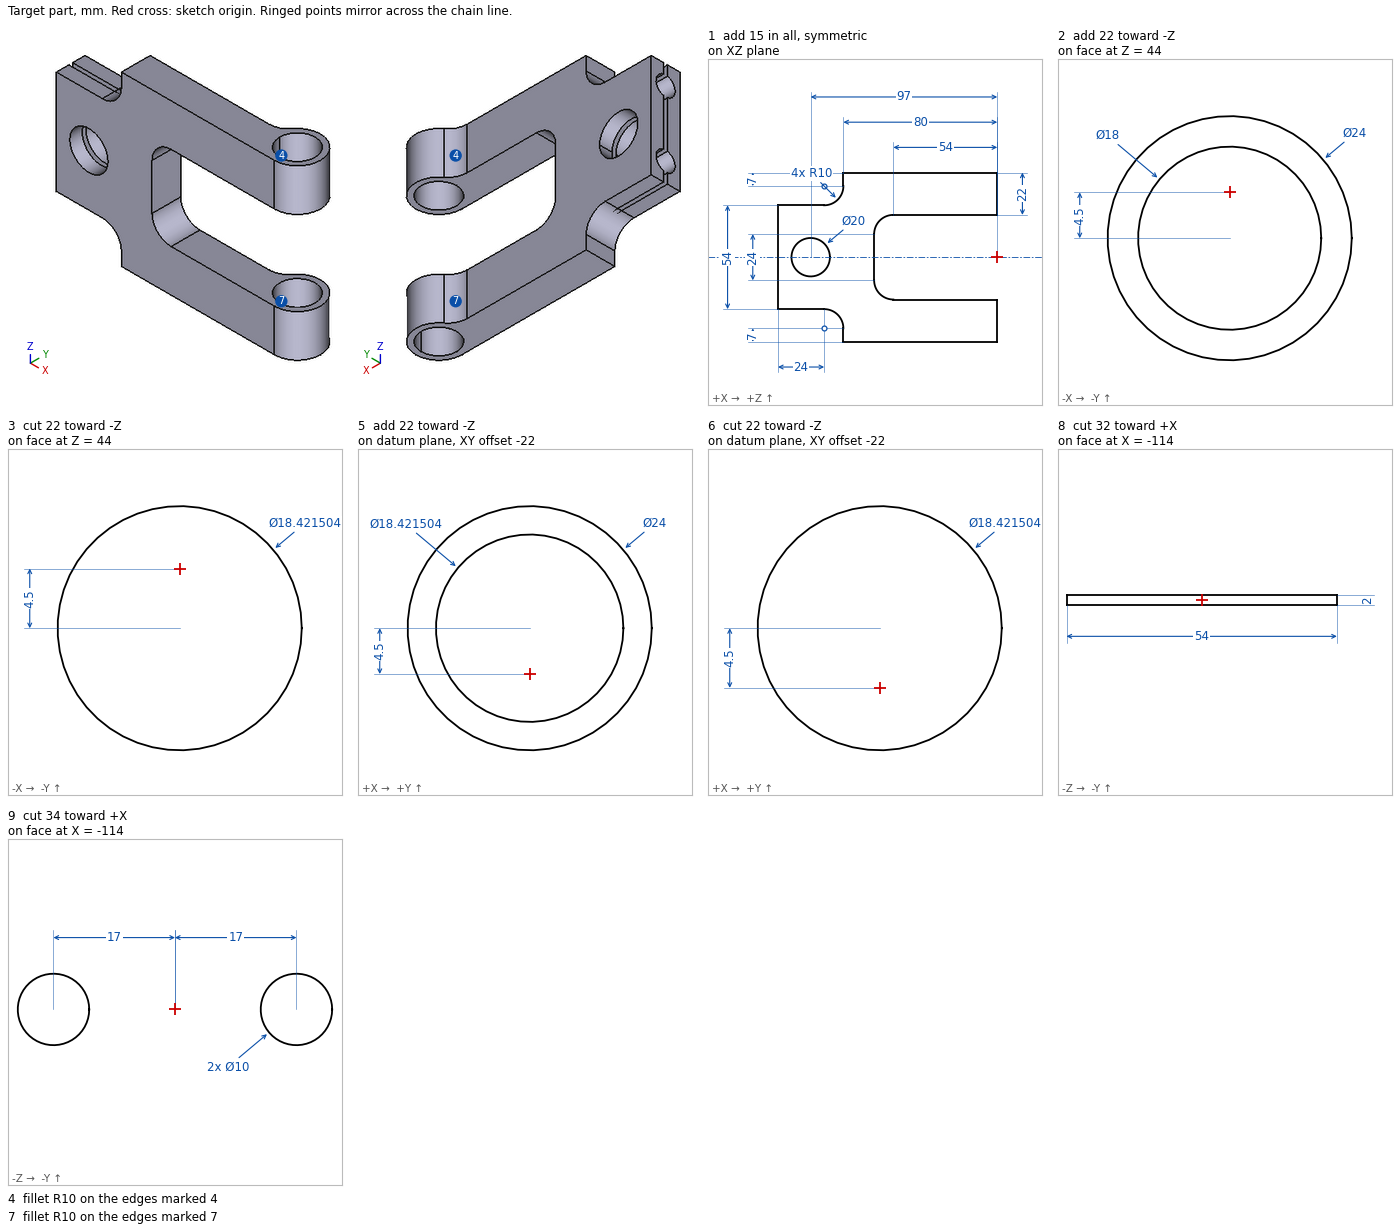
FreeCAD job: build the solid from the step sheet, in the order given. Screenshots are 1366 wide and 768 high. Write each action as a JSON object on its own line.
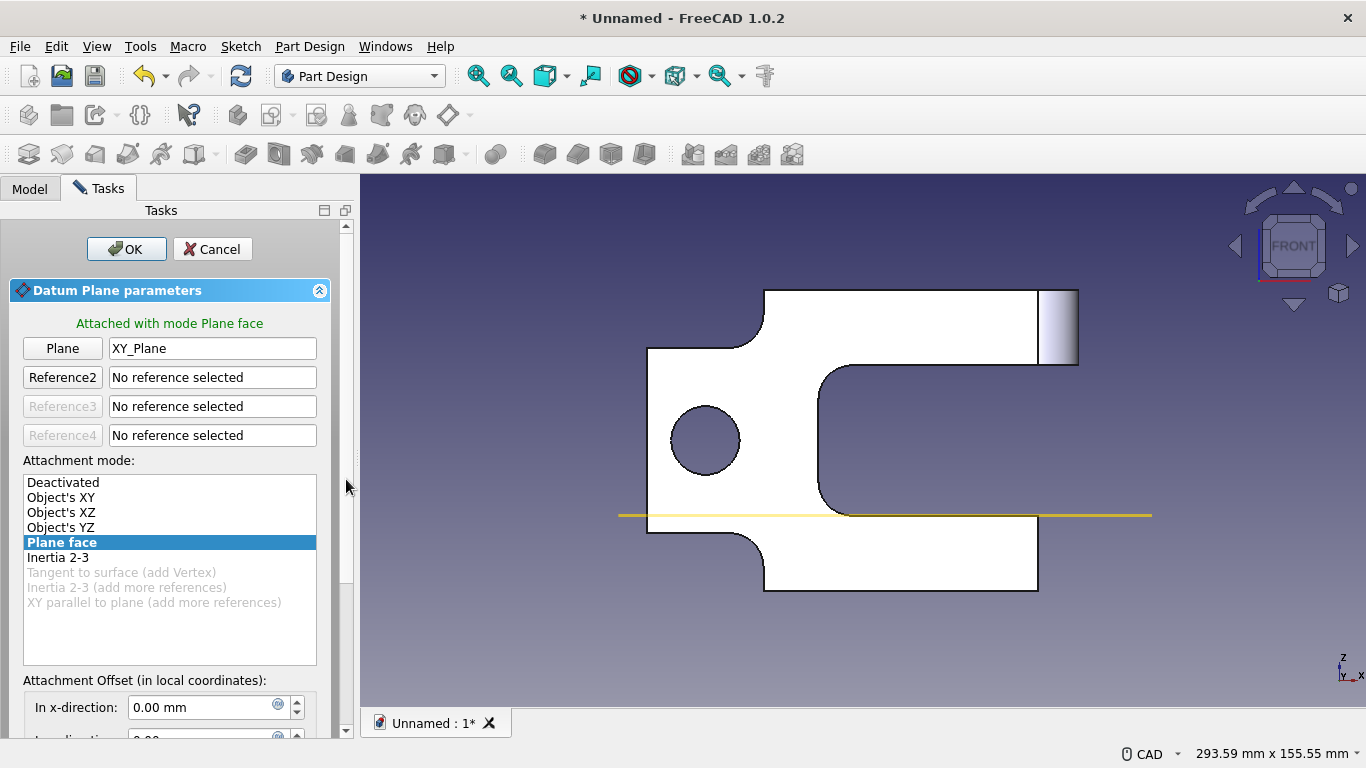
{"action": "left_click", "coordinate": [127, 249]}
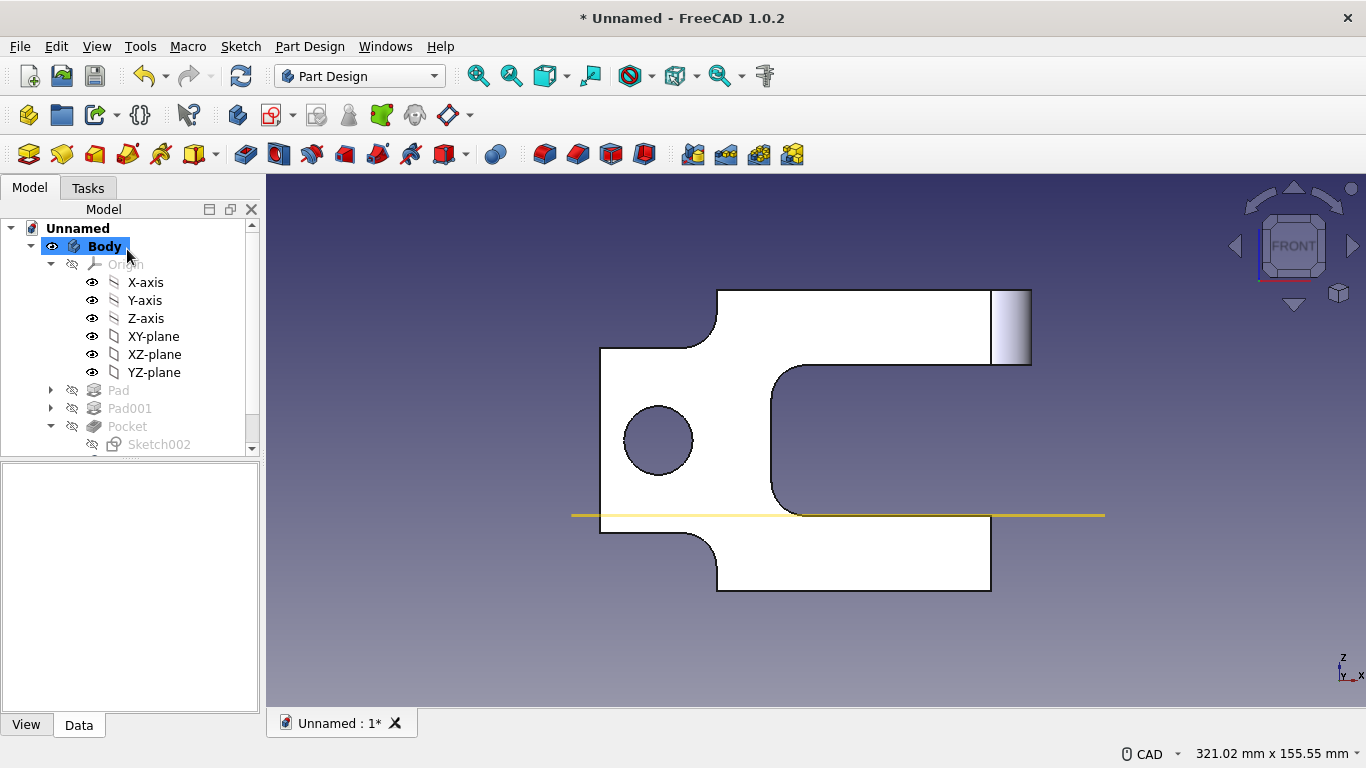
{"action": "scroll", "coordinate": [101, 332], "scroll_direction": "down", "scroll_amount": 3}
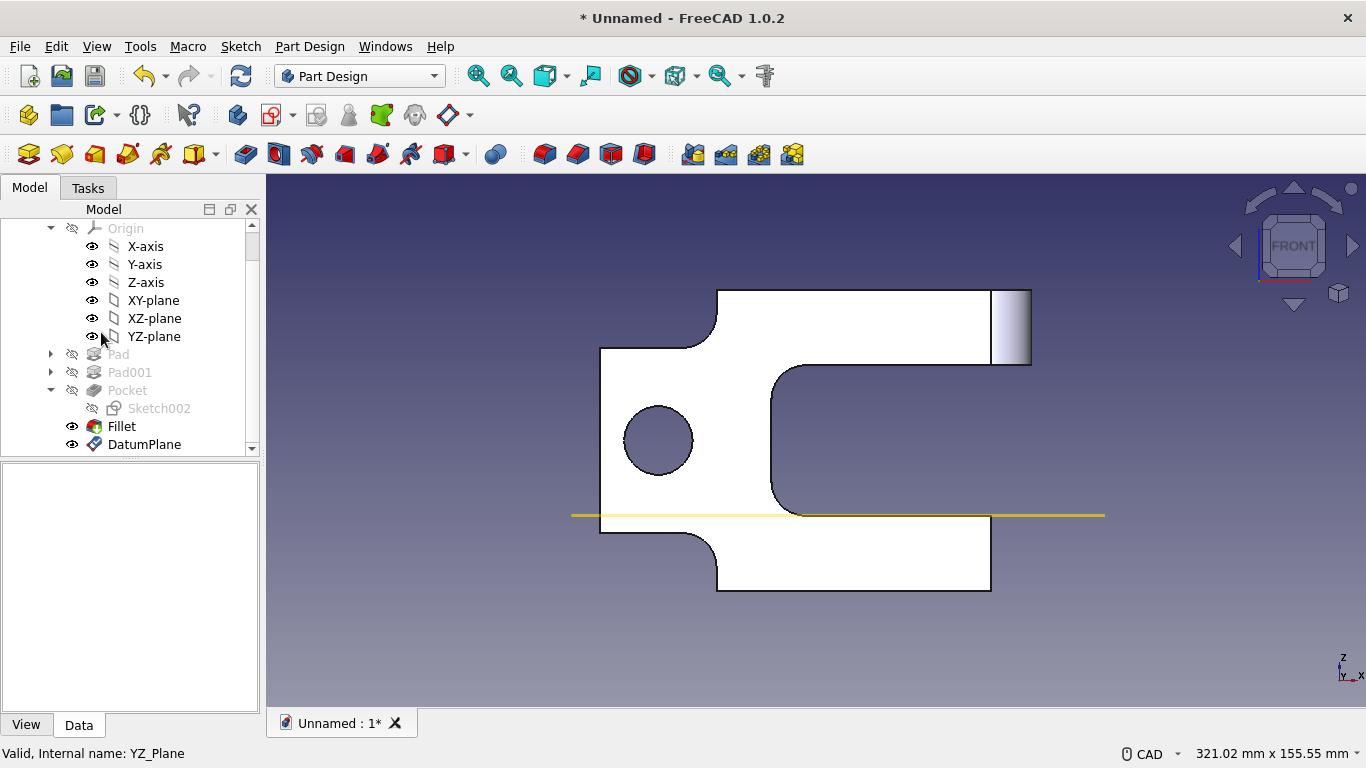
{"action": "left_click", "coordinate": [117, 444]}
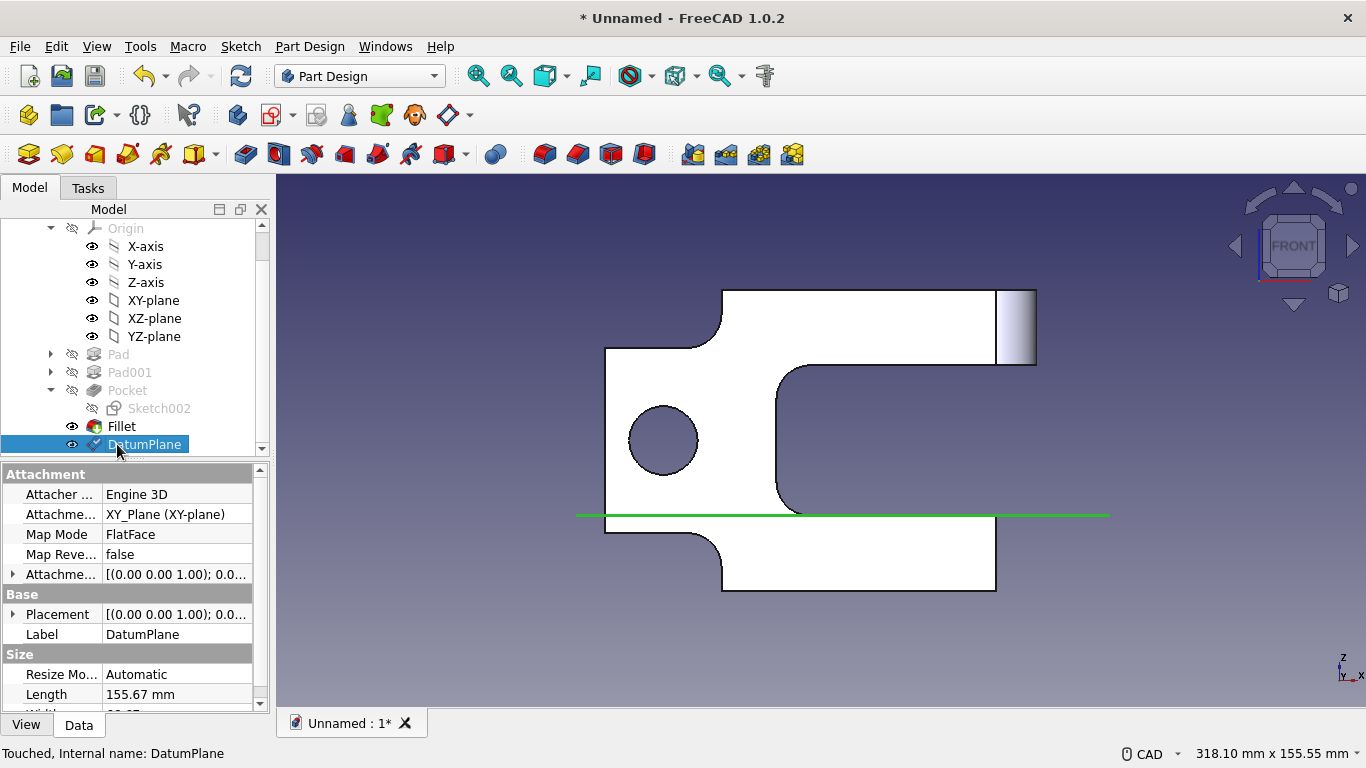
{"action": "left_click", "coordinate": [270, 116]}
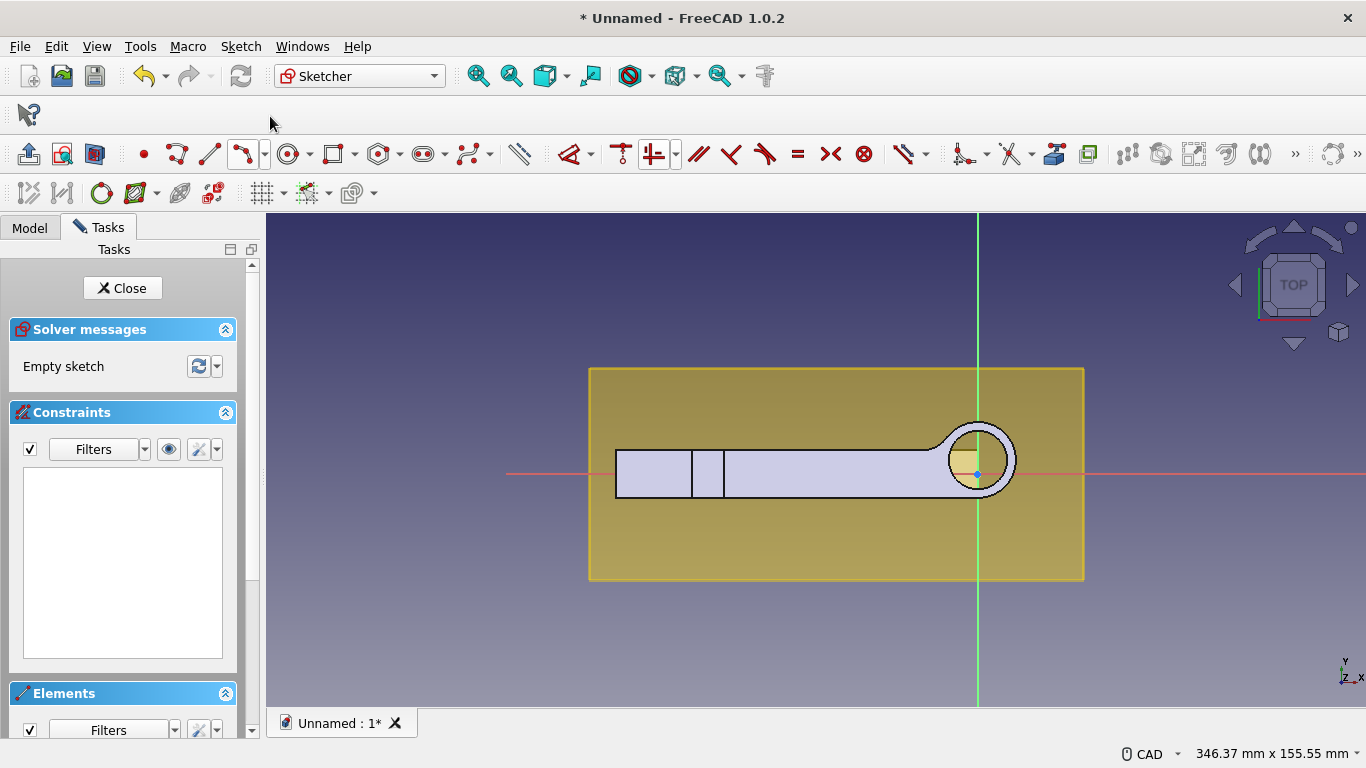
{"action": "left_click", "coordinate": [95, 154]}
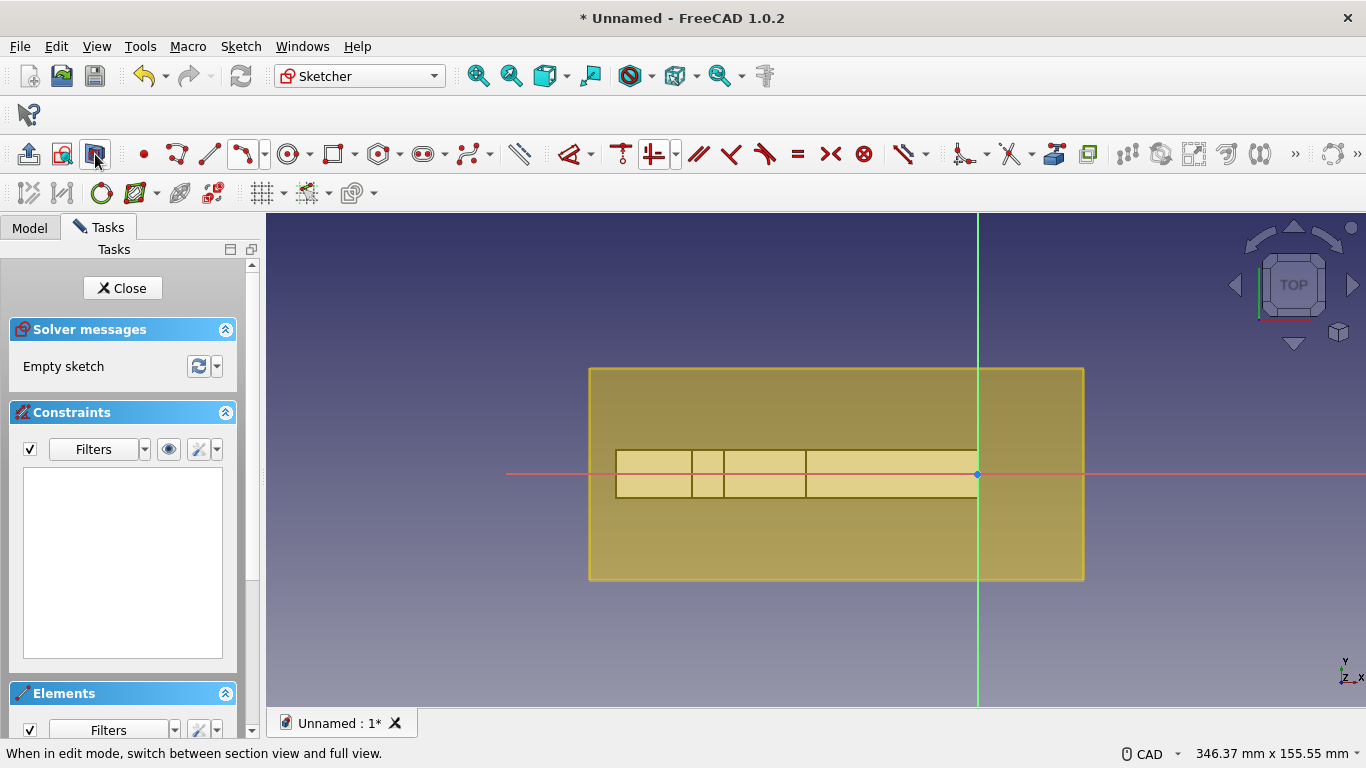
{"action": "scroll", "coordinate": [1053, 460], "scroll_direction": "up", "scroll_amount": 7}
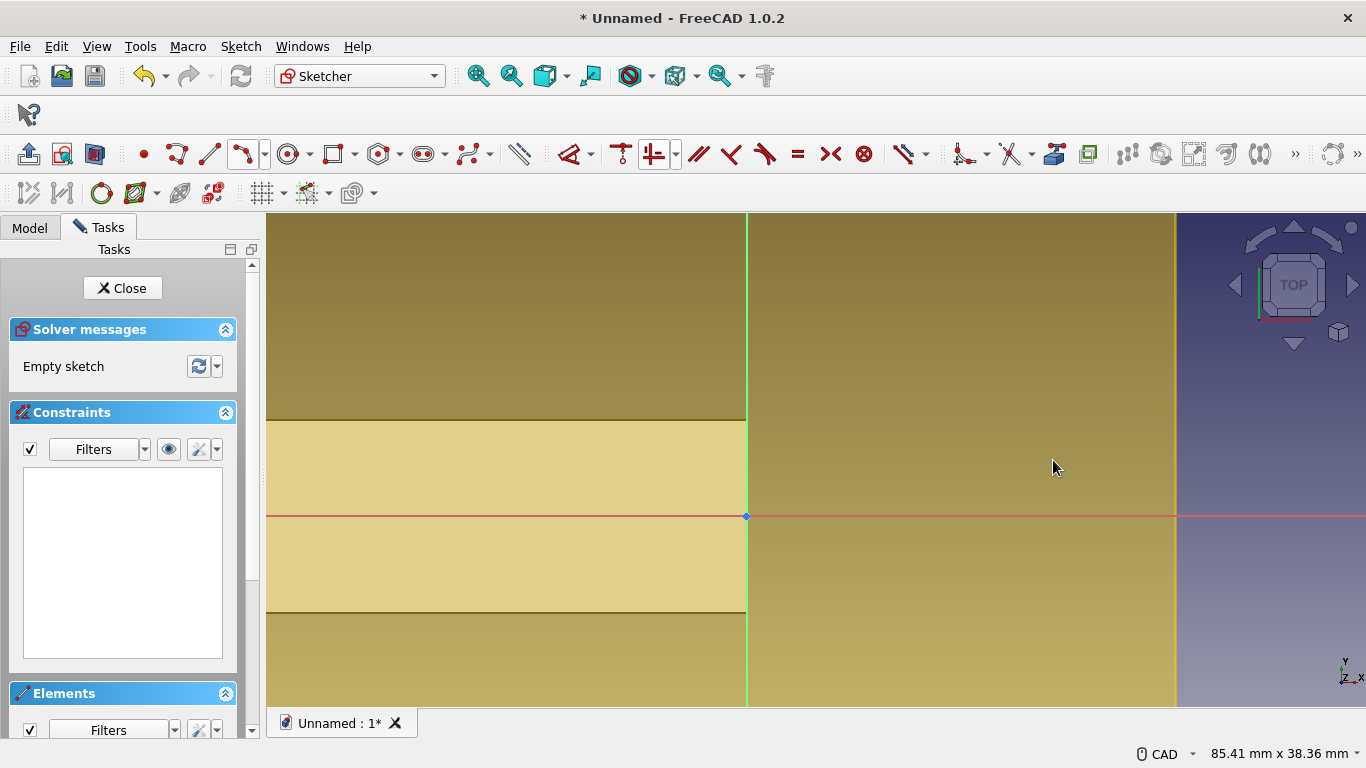
{"action": "left_click", "coordinate": [288, 154]}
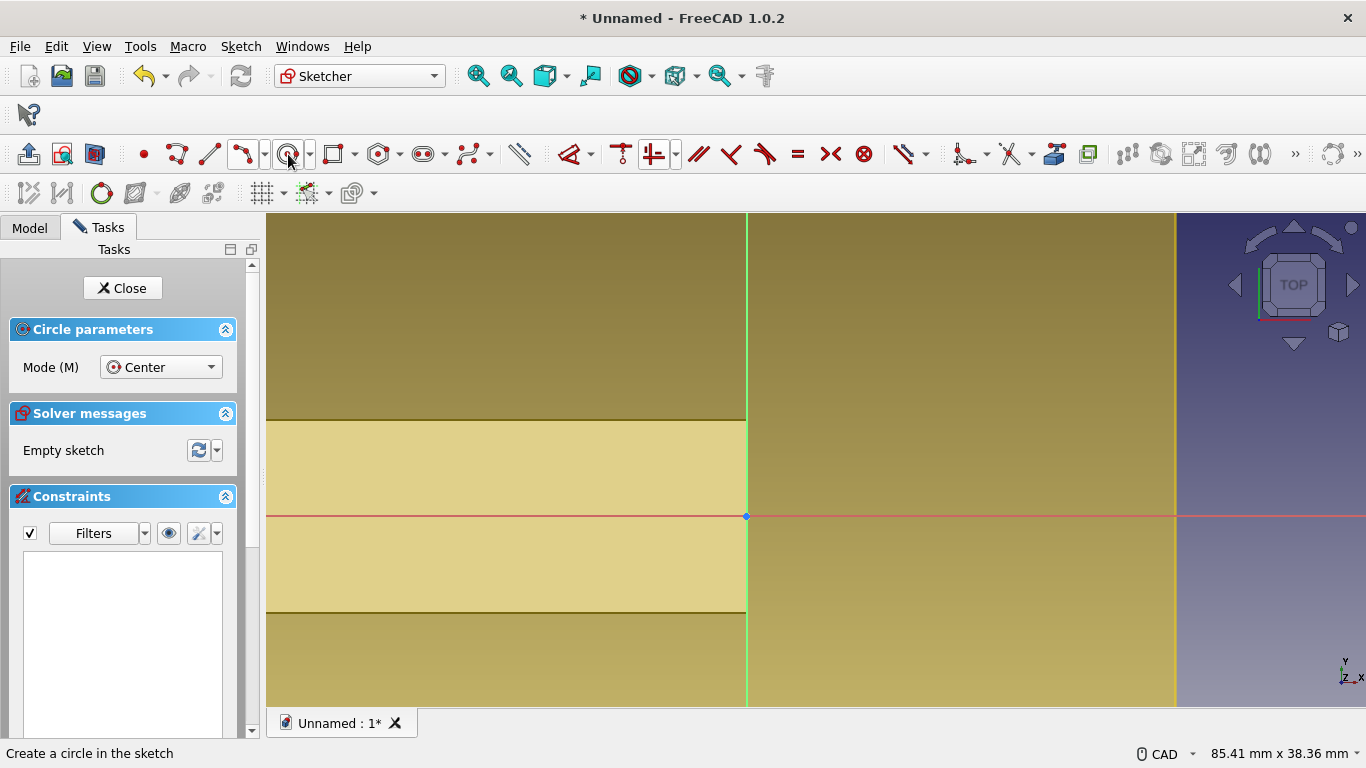
{"action": "left_click", "coordinate": [747, 458]}
{"action": "left_click", "coordinate": [856, 349]}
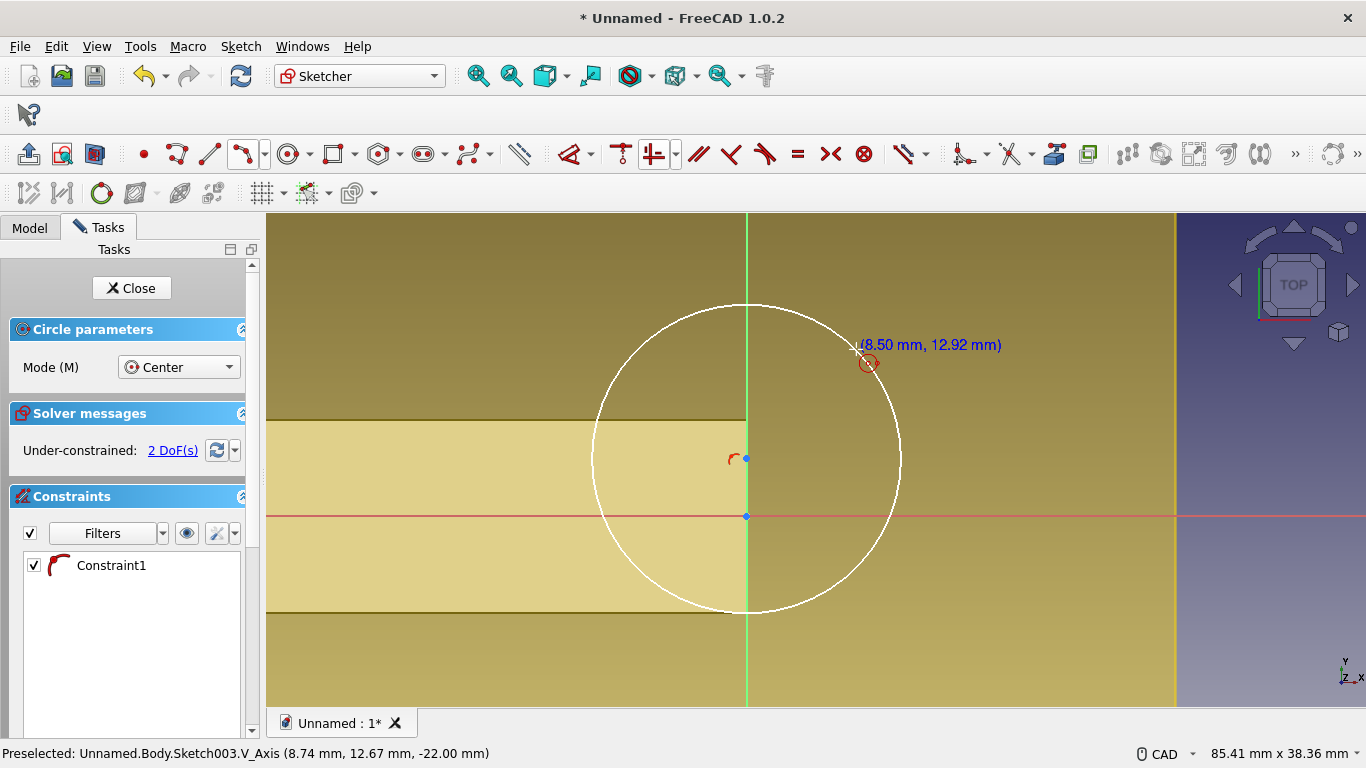
{"action": "left_click", "coordinate": [747, 459]}
{"action": "left_click", "coordinate": [830, 375]}
{"action": "key", "text": "Escape"}